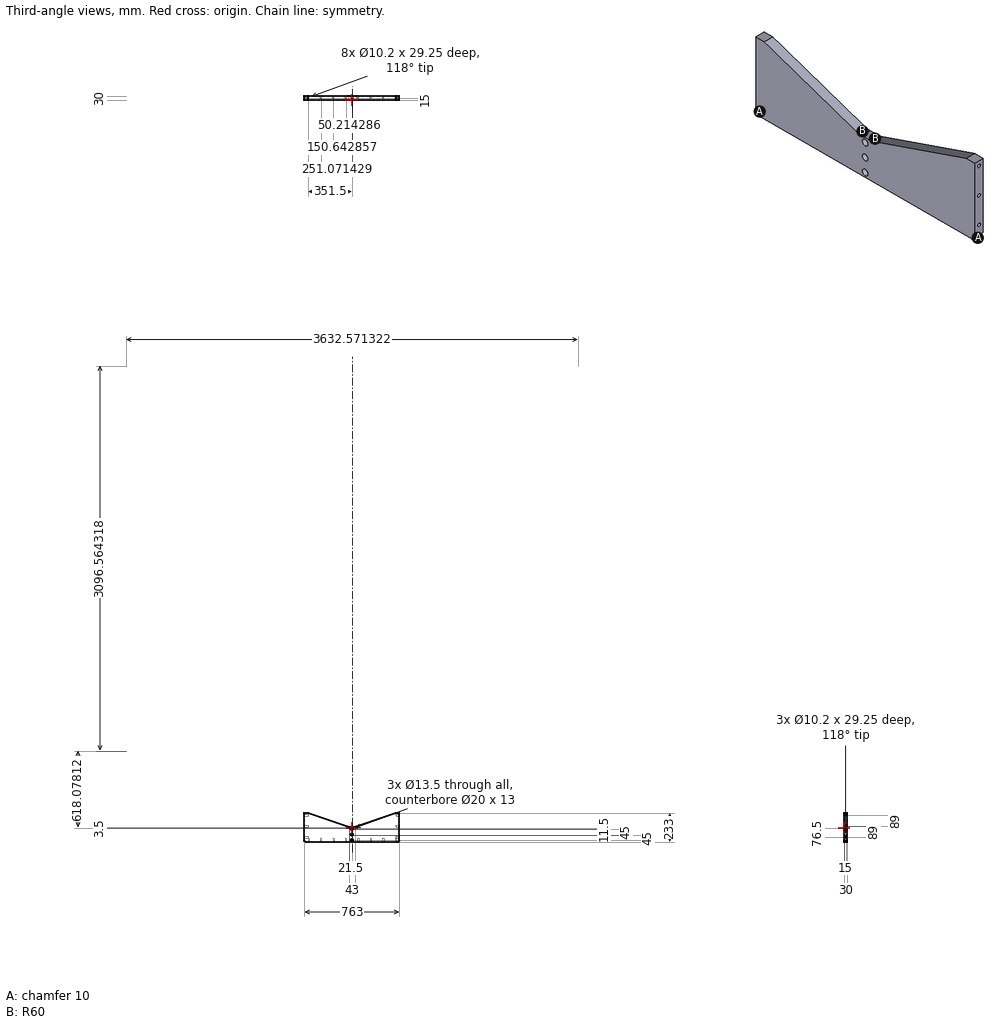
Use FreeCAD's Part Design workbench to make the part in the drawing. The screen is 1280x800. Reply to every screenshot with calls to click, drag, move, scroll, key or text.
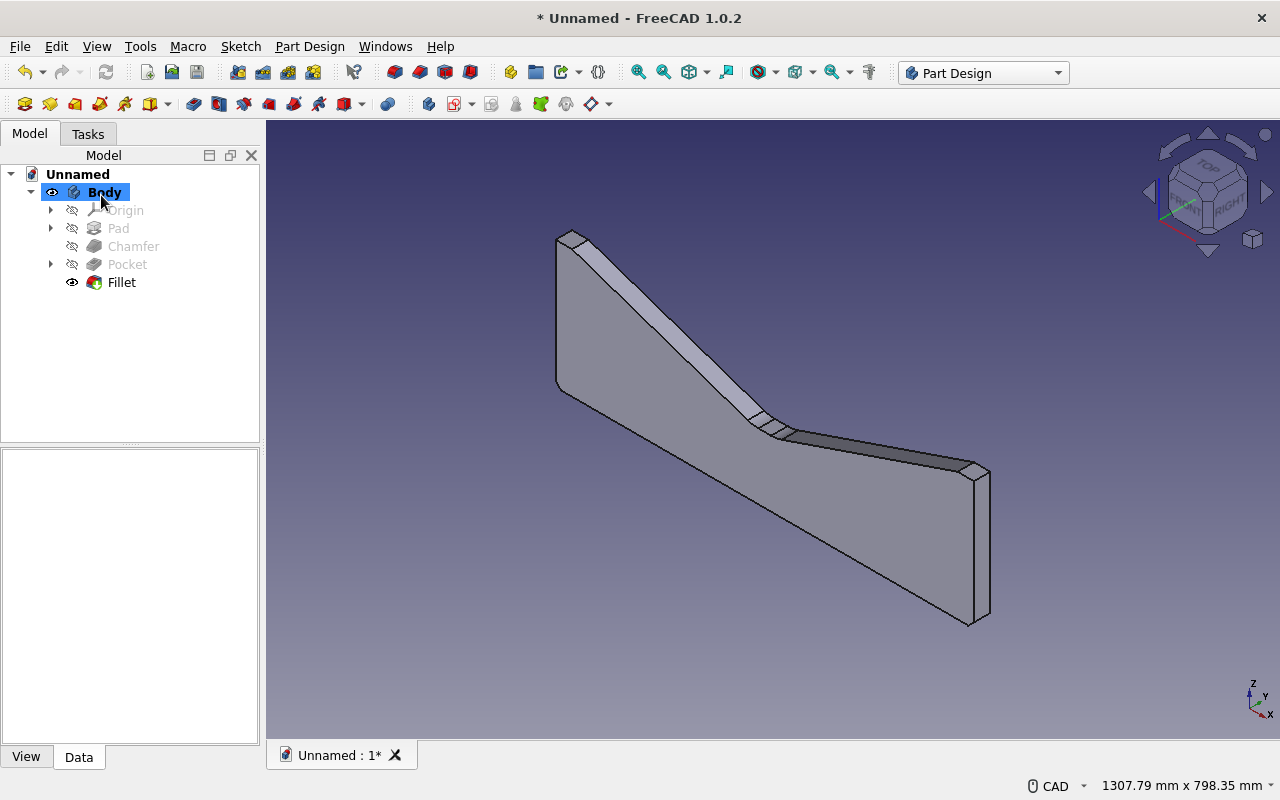
click(884, 523)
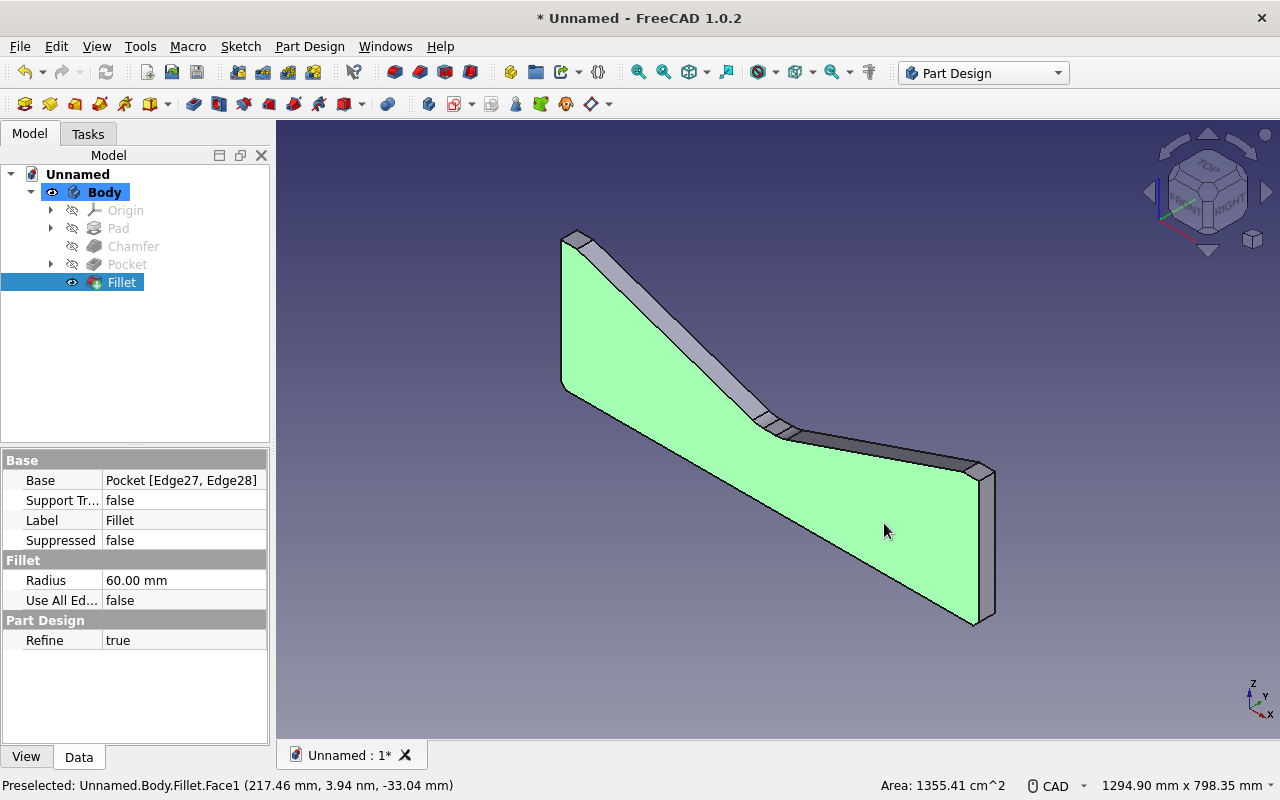
click(454, 104)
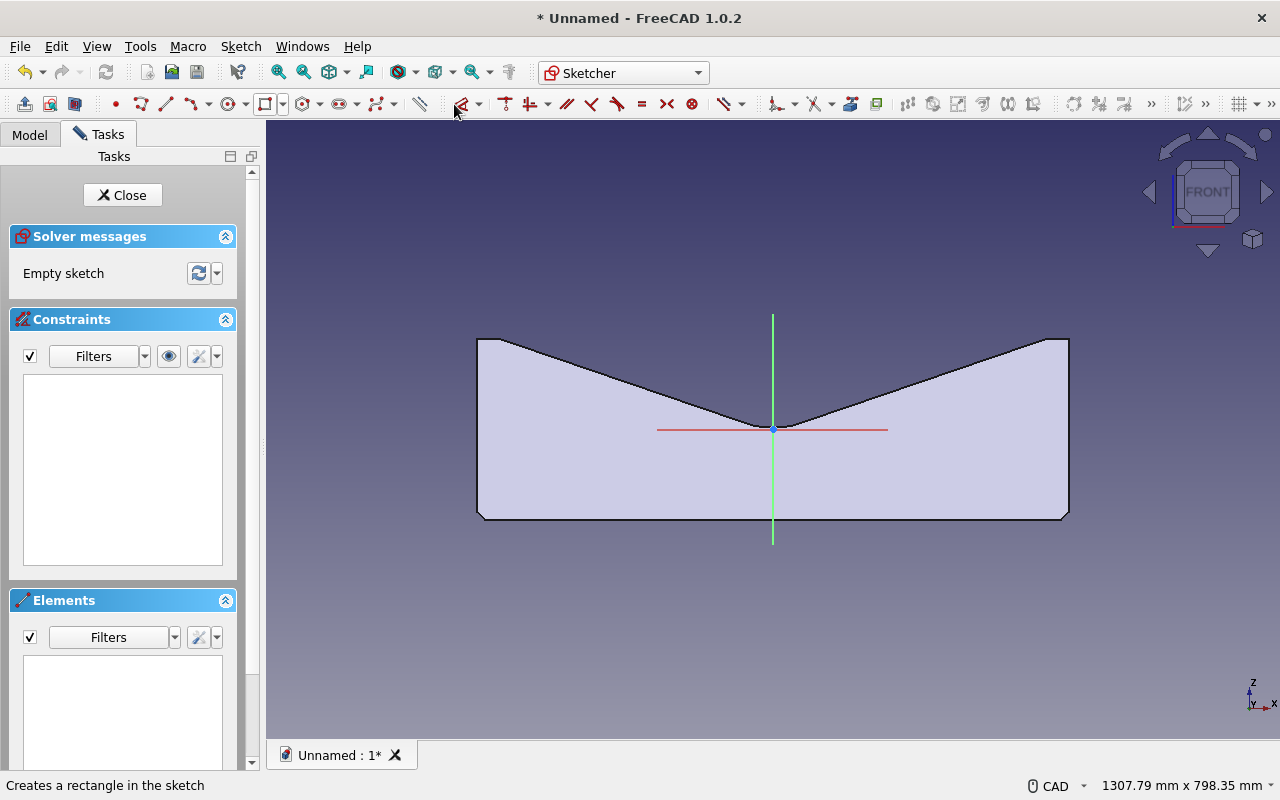
scroll(790, 482, up, 8)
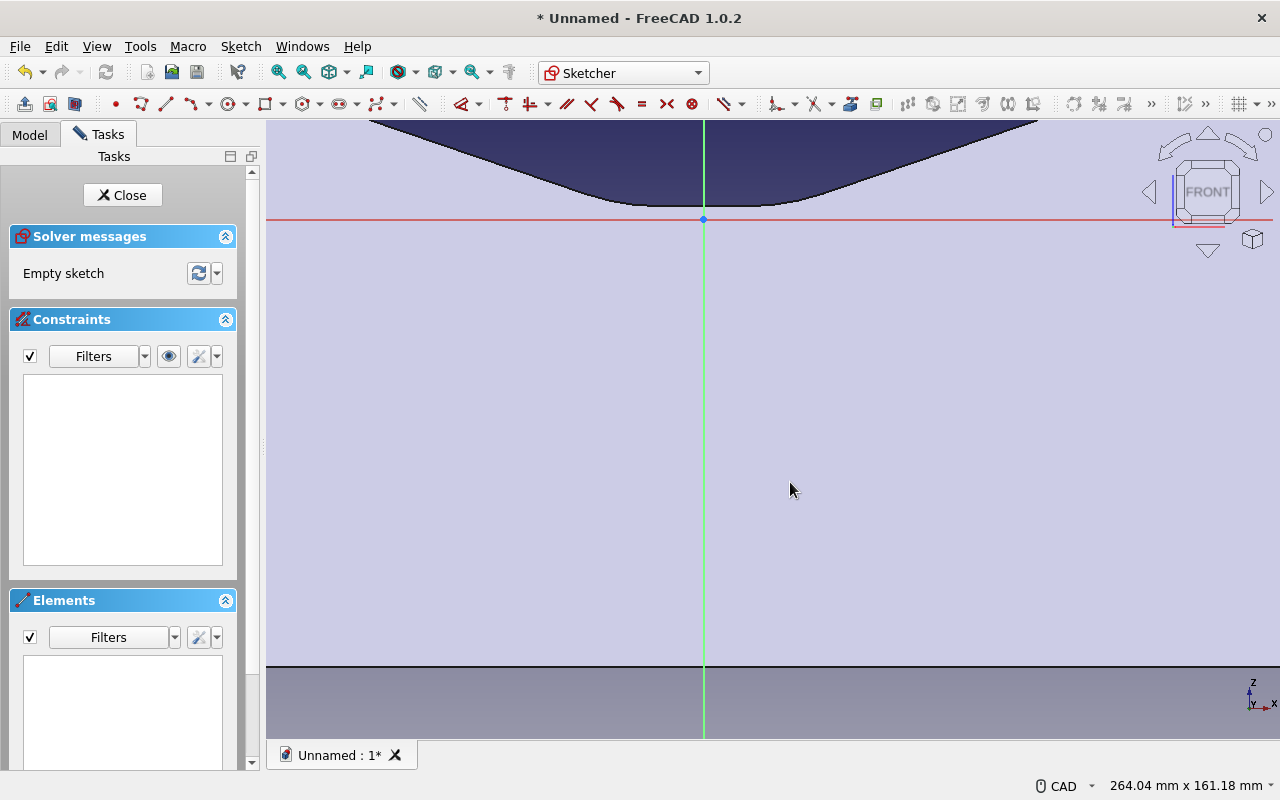
key(g)
key(c)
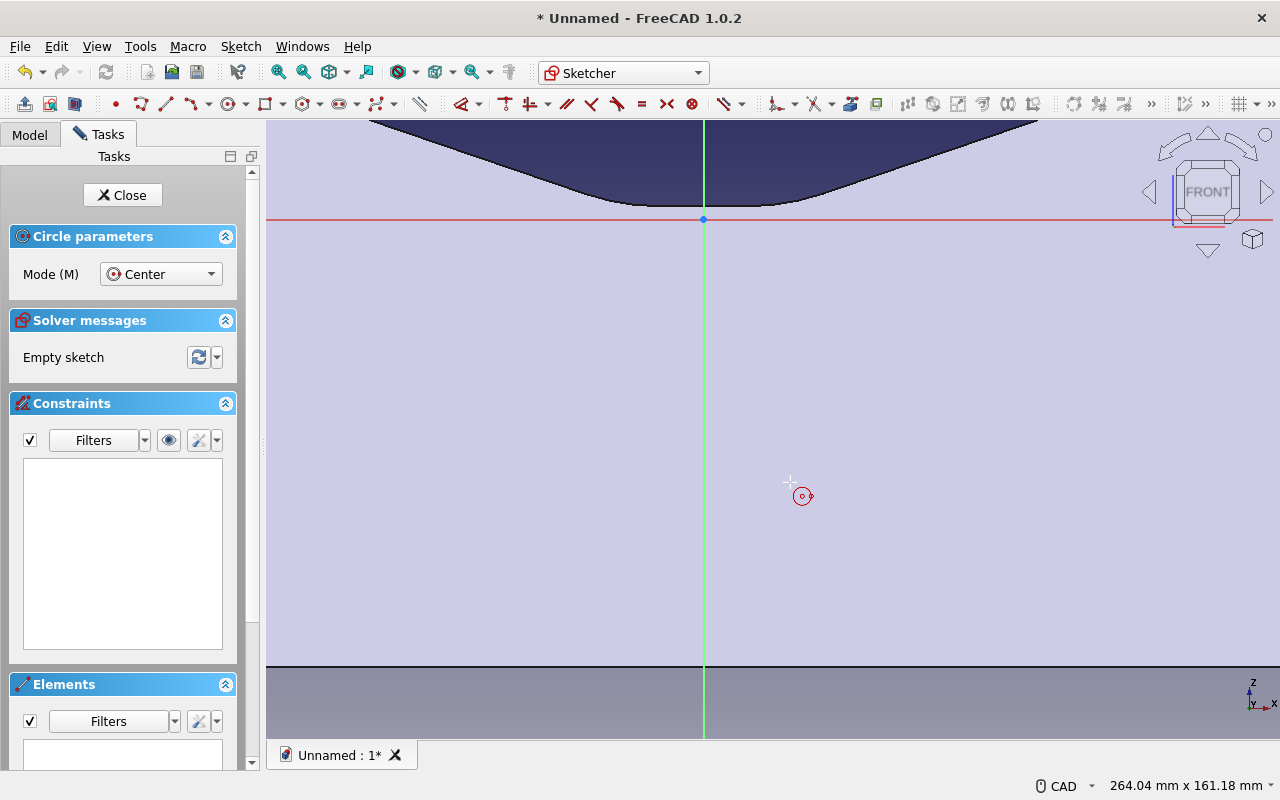
click(704, 264)
click(722, 245)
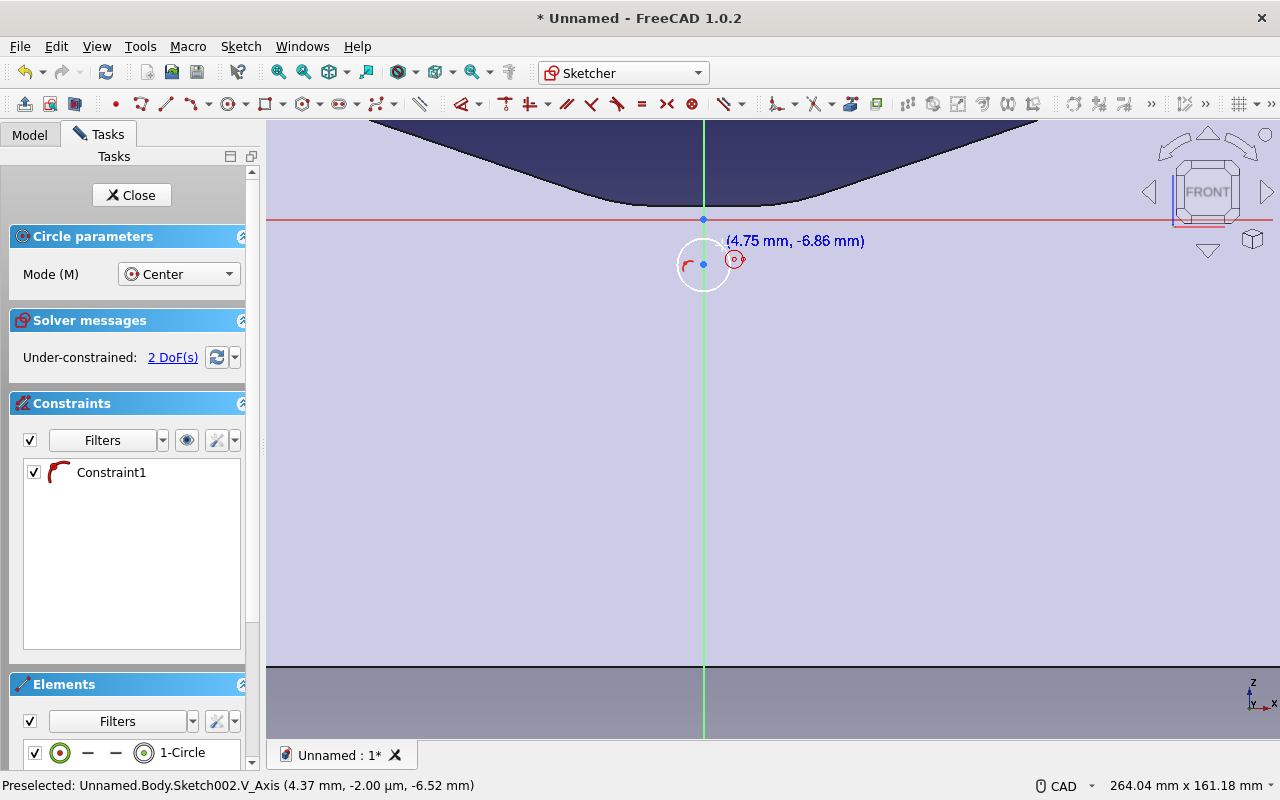
click(704, 437)
click(722, 418)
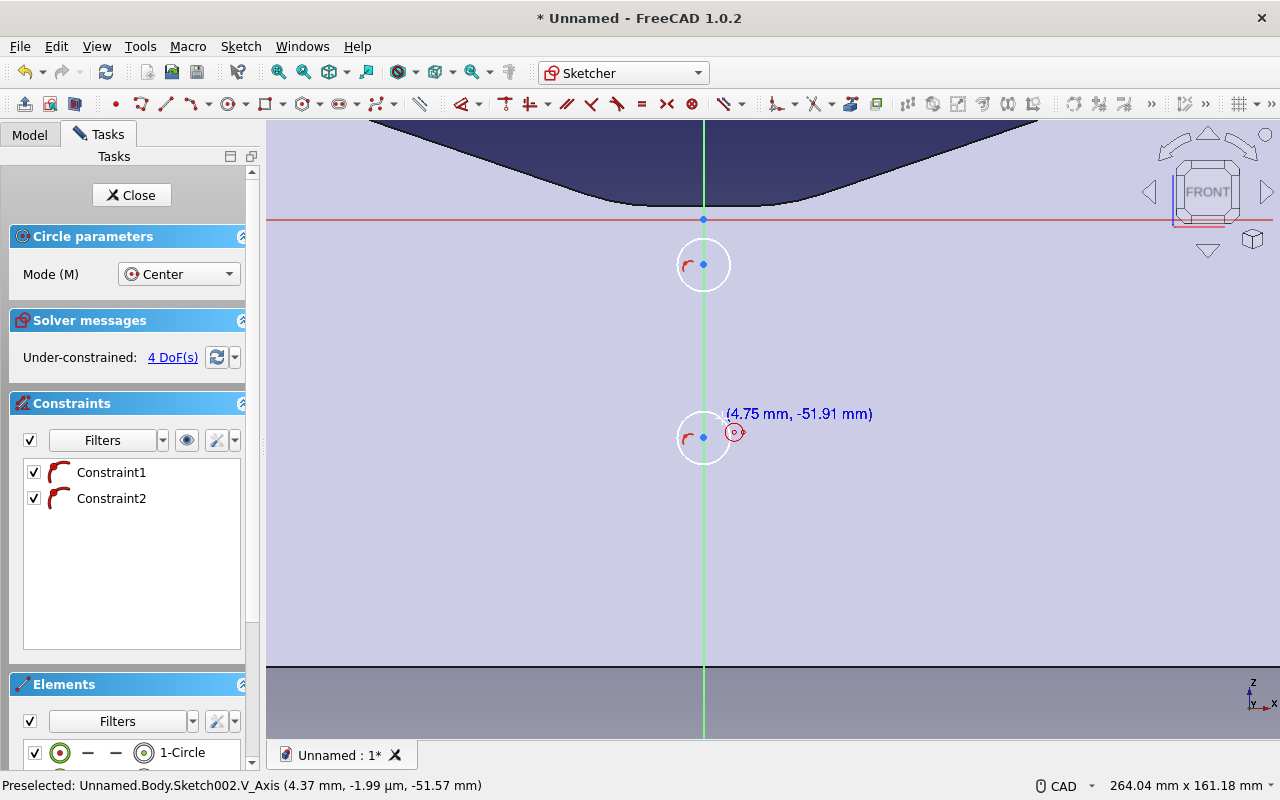
click(704, 609)
click(722, 591)
key(Escape)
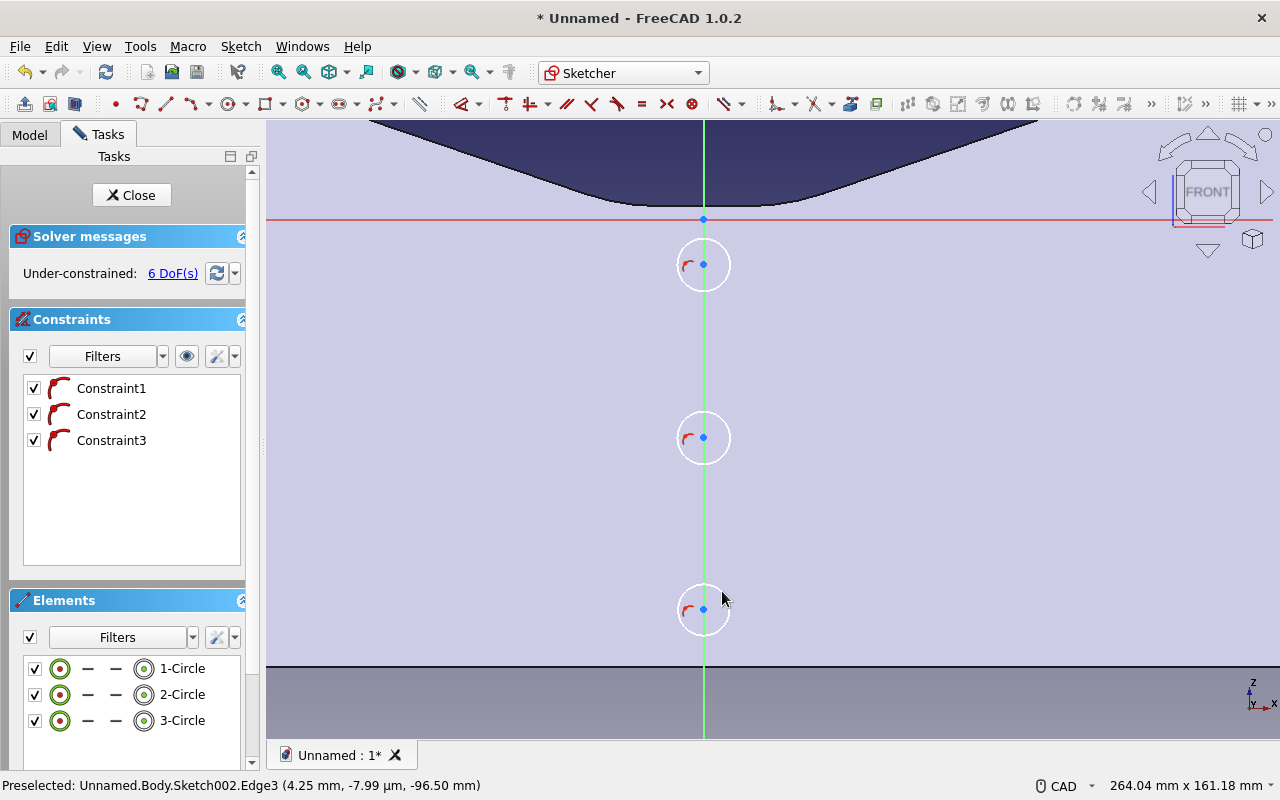
click(722, 246)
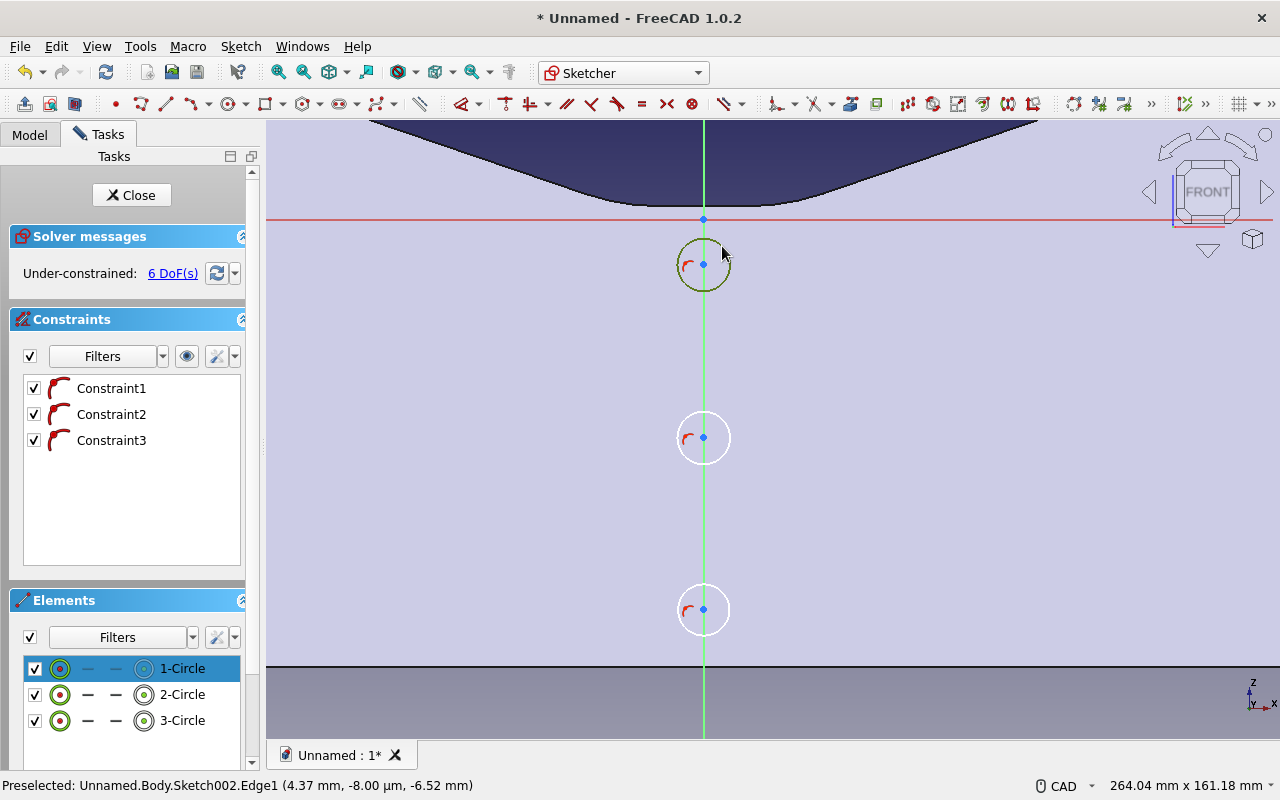
click(722, 419)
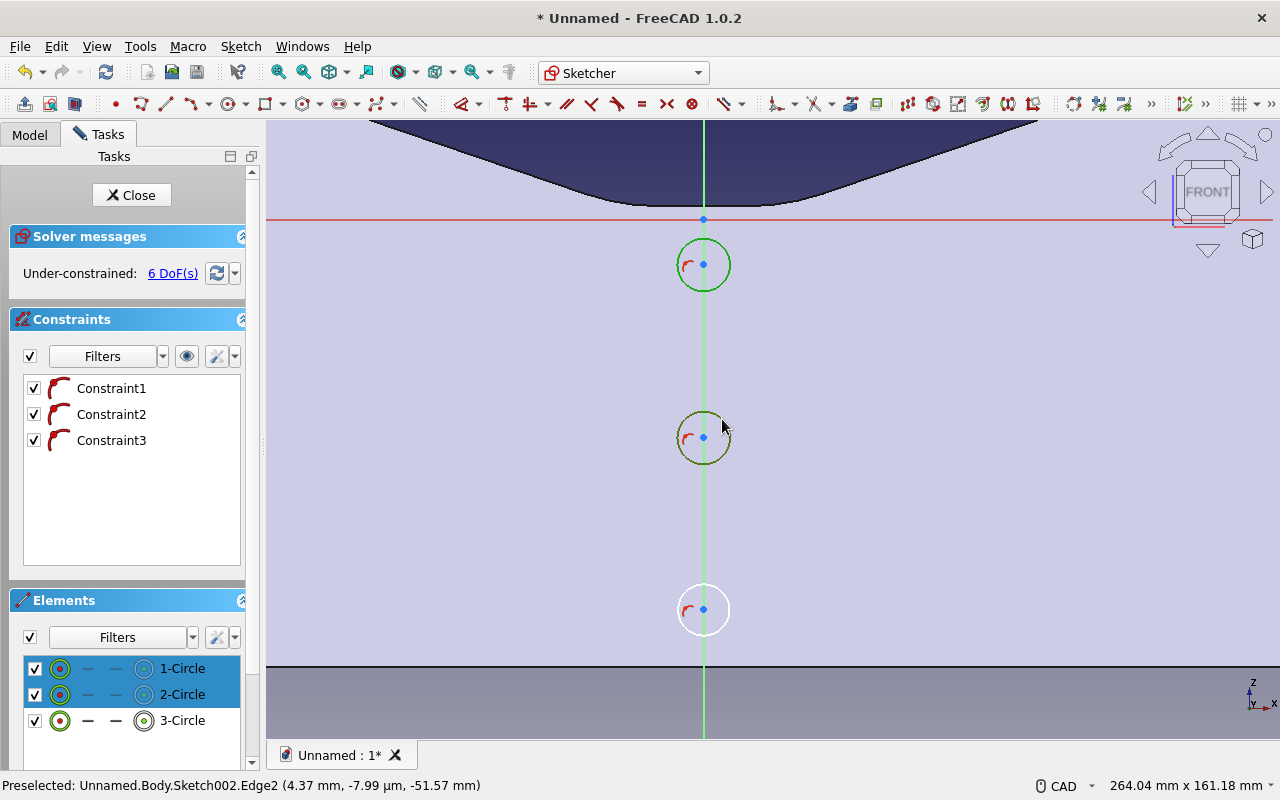
click(722, 592)